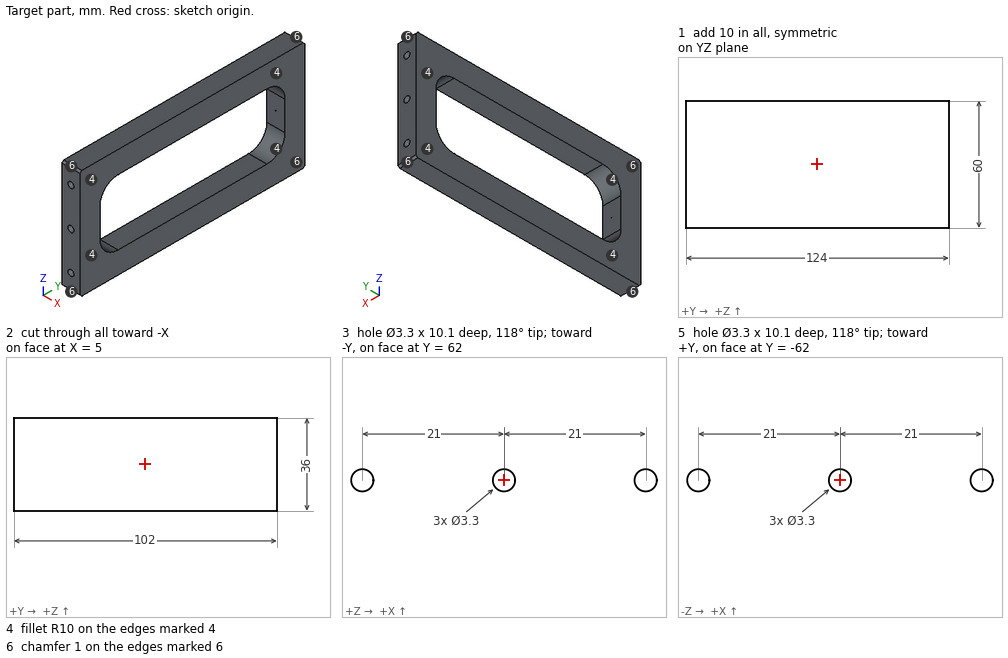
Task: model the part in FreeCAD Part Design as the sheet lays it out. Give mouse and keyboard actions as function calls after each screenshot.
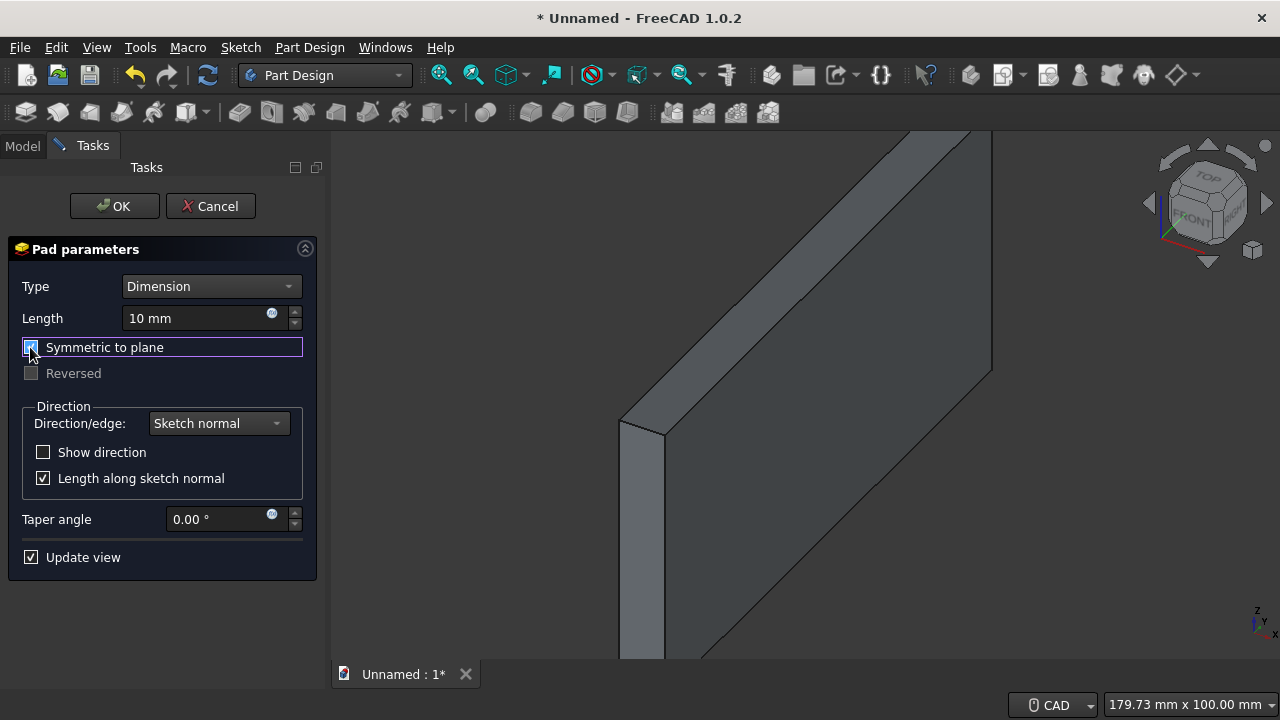
click(115, 206)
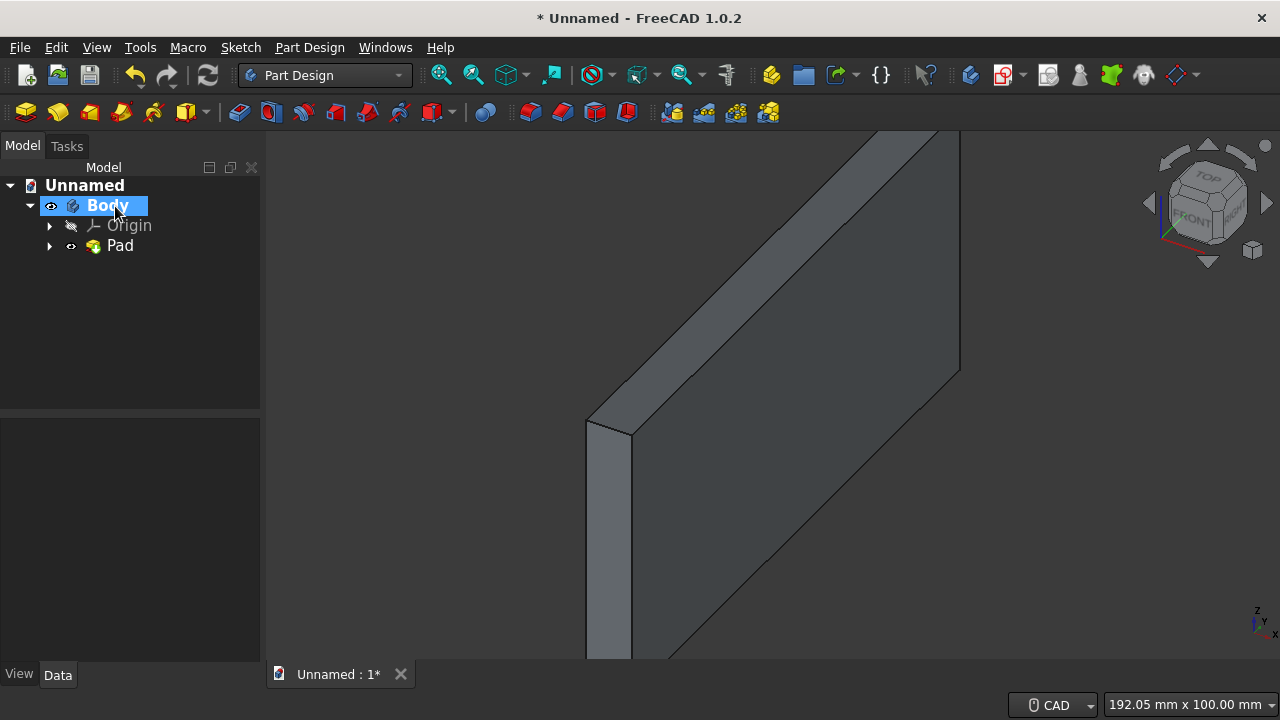
click(442, 76)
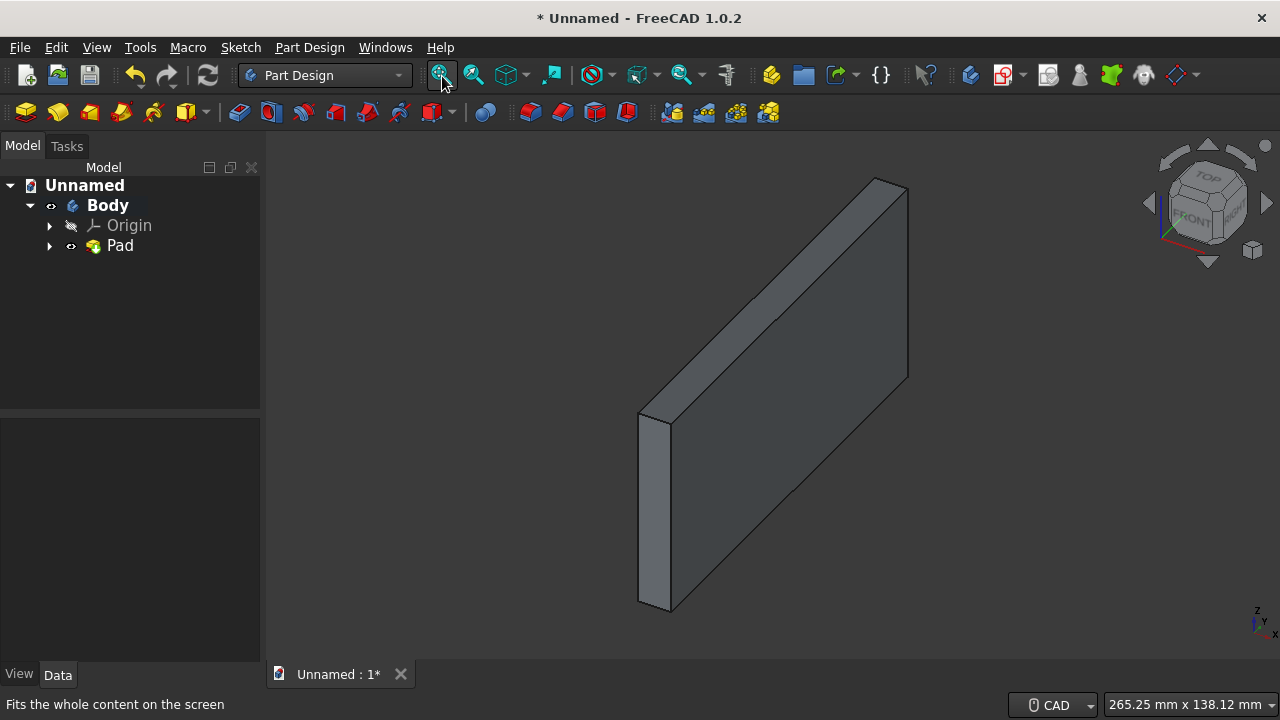
click(790, 399)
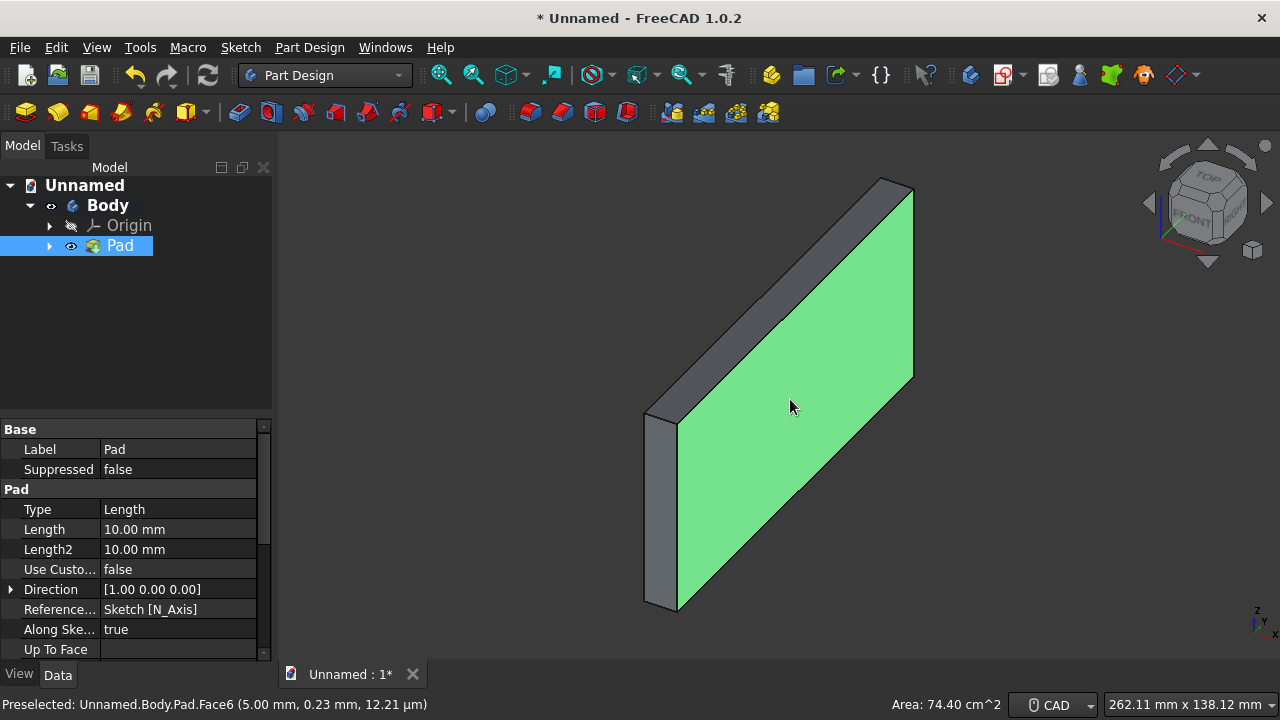
click(1004, 76)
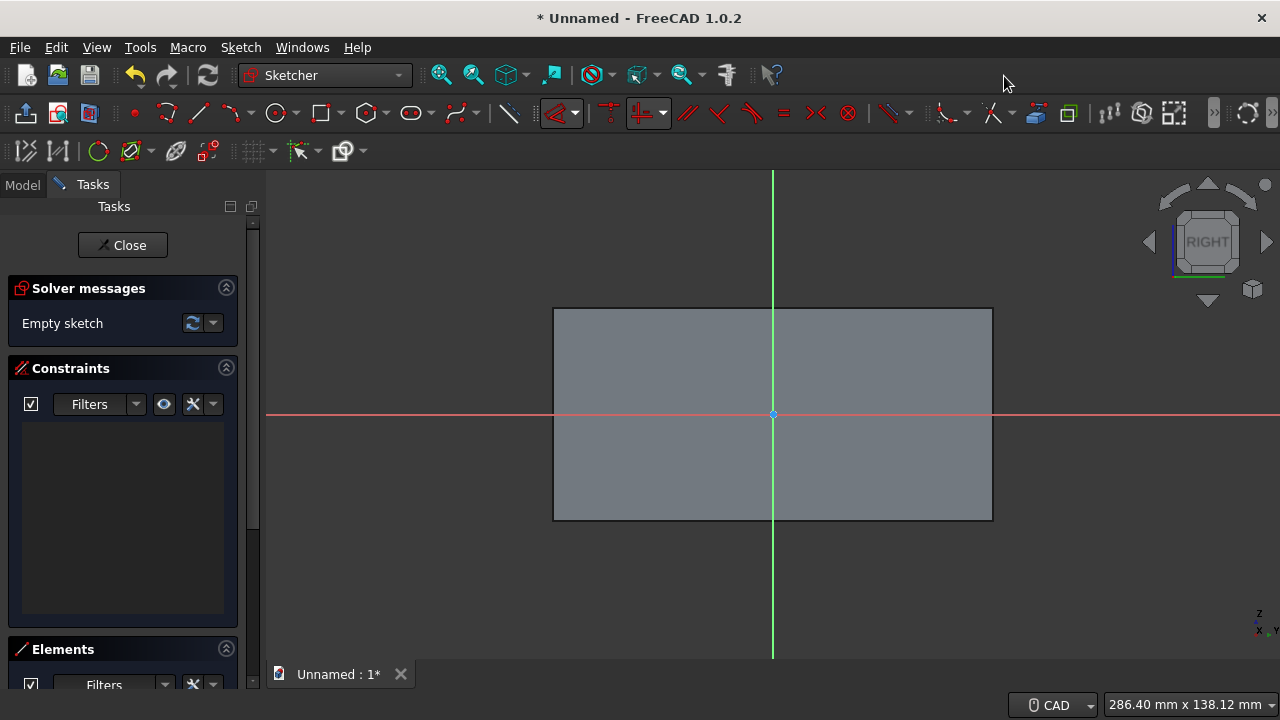
scroll(912, 414, up, 2)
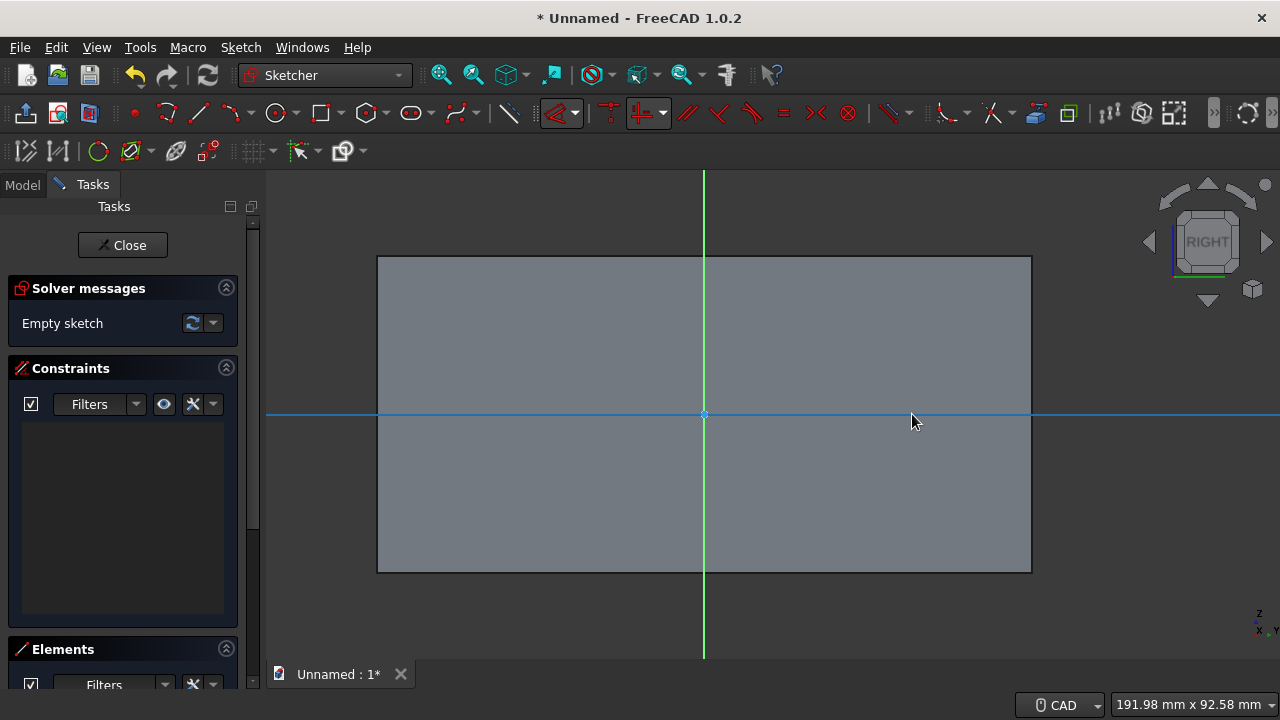
key(g)
key(v)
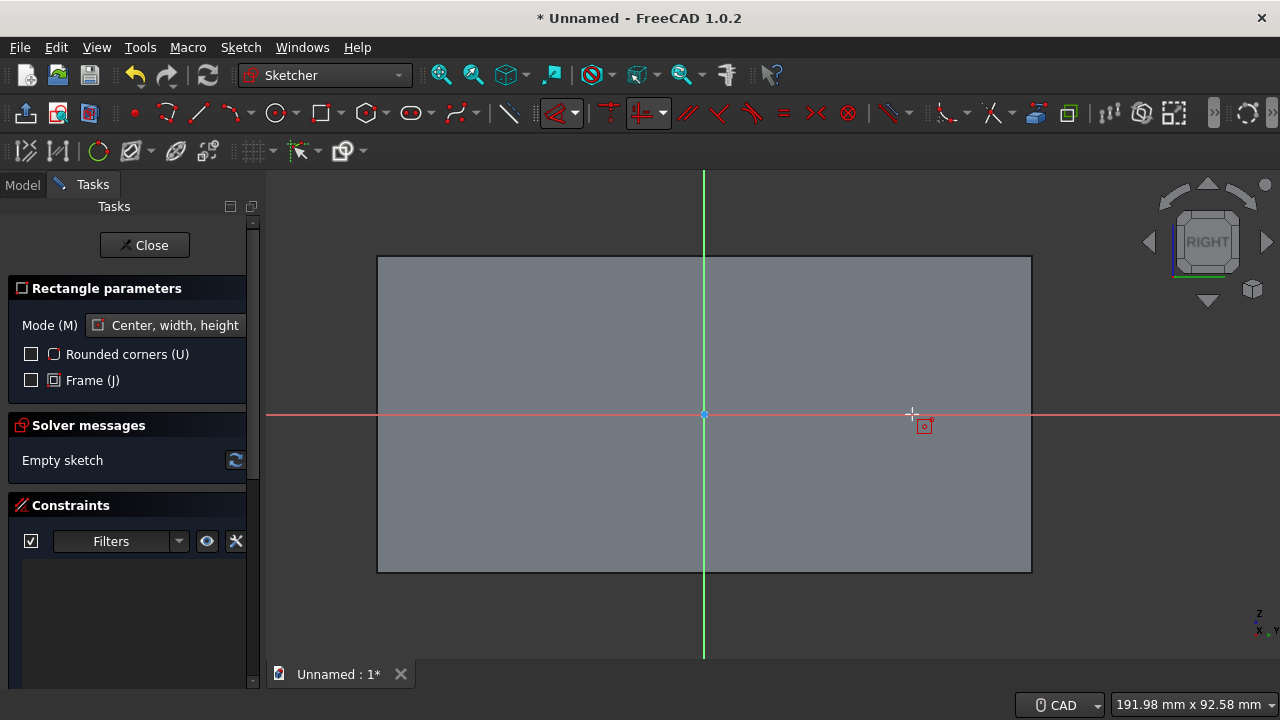
click(704, 414)
move(974, 319)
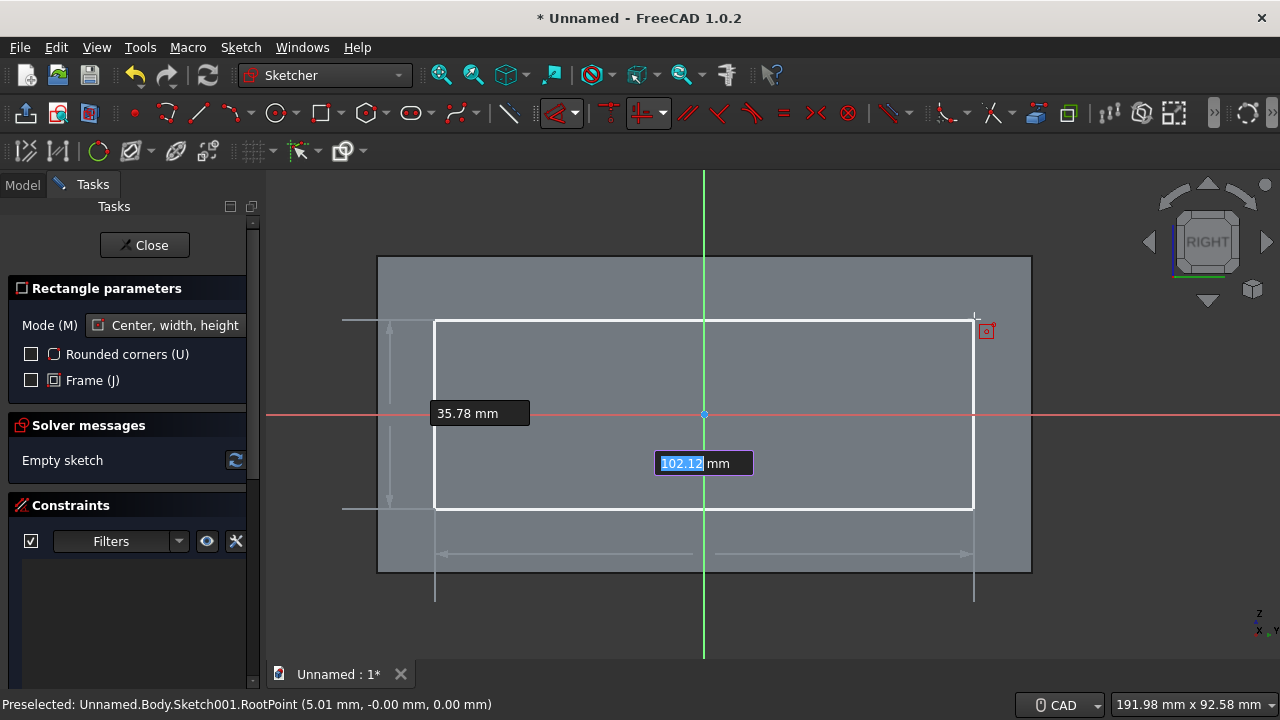
text(102)
key(Tab)
text(36)
key(Return)
key(Escape)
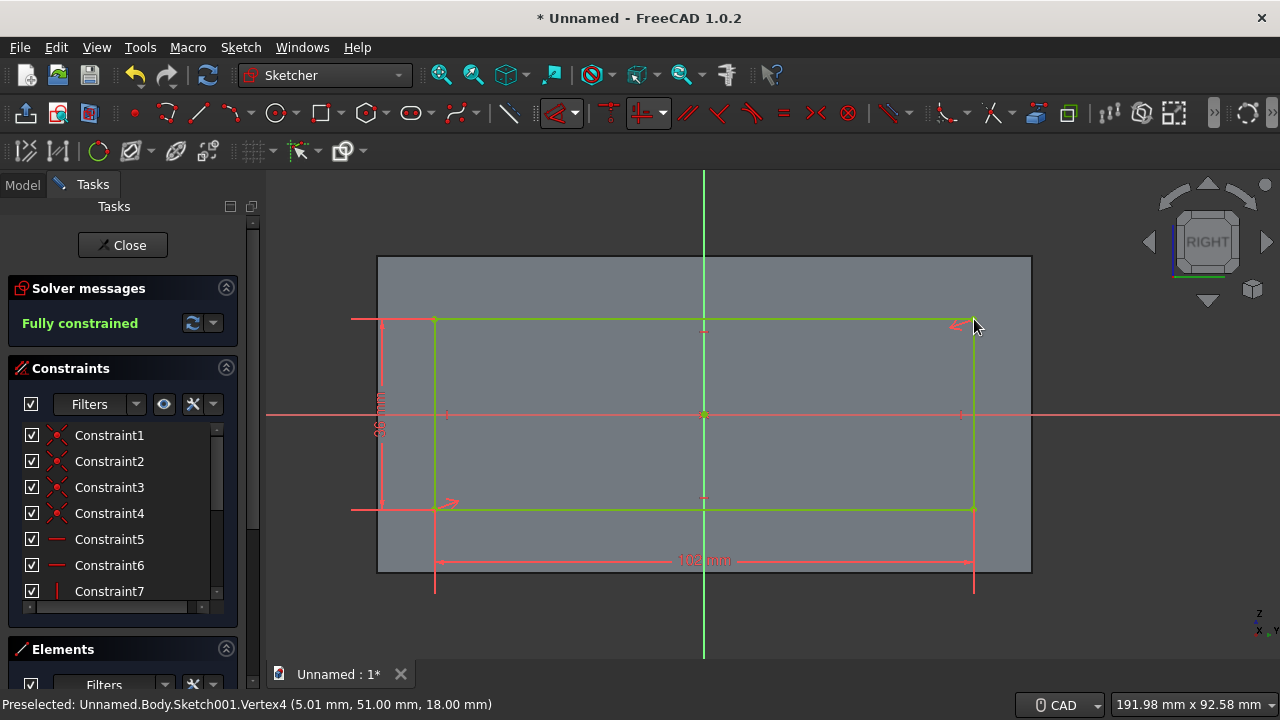
click(123, 245)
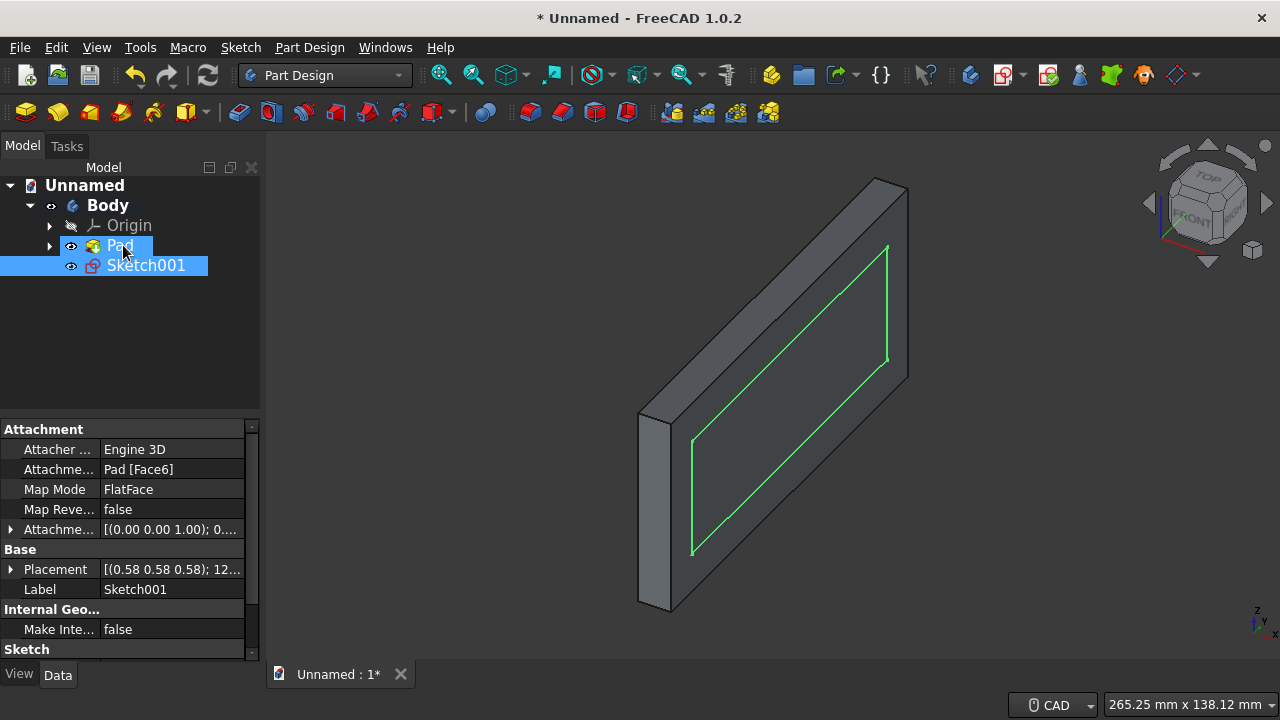
click(240, 112)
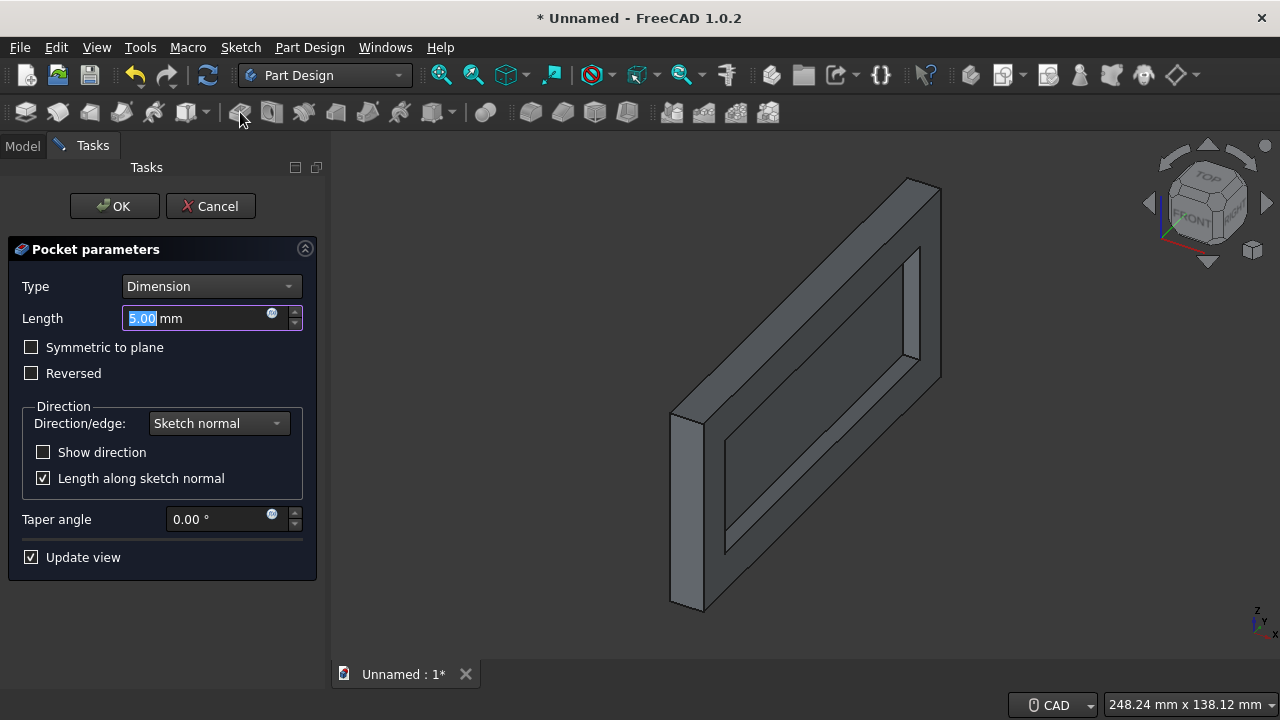
click(212, 286)